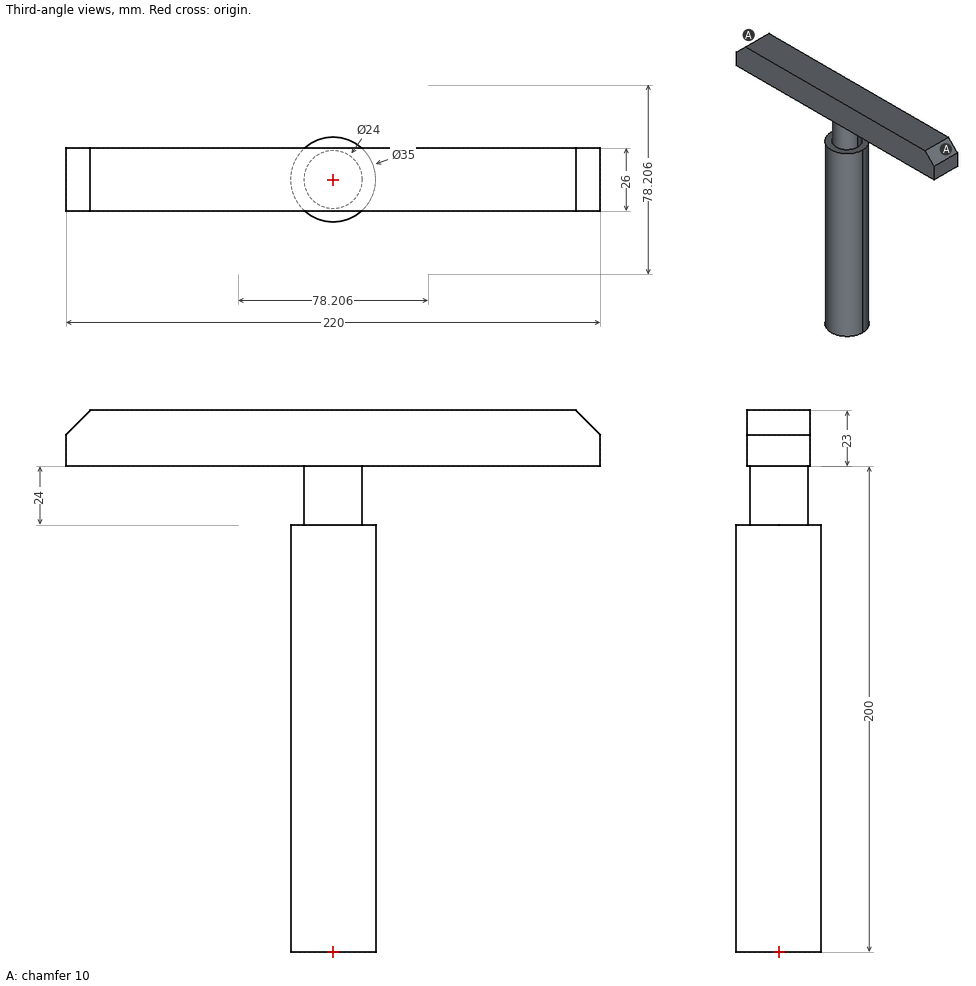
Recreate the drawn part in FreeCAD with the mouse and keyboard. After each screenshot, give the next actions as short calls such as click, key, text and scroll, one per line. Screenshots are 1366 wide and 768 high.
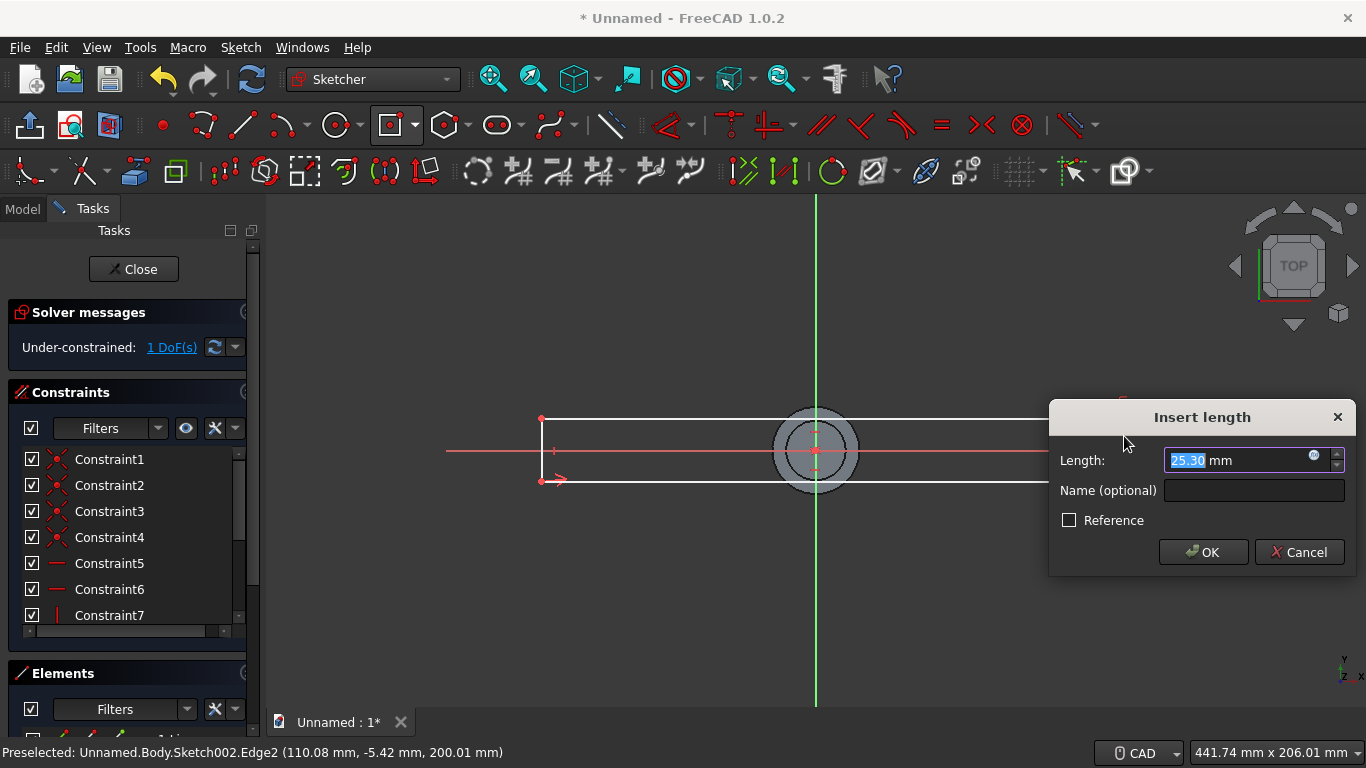
text(26)
key(Return)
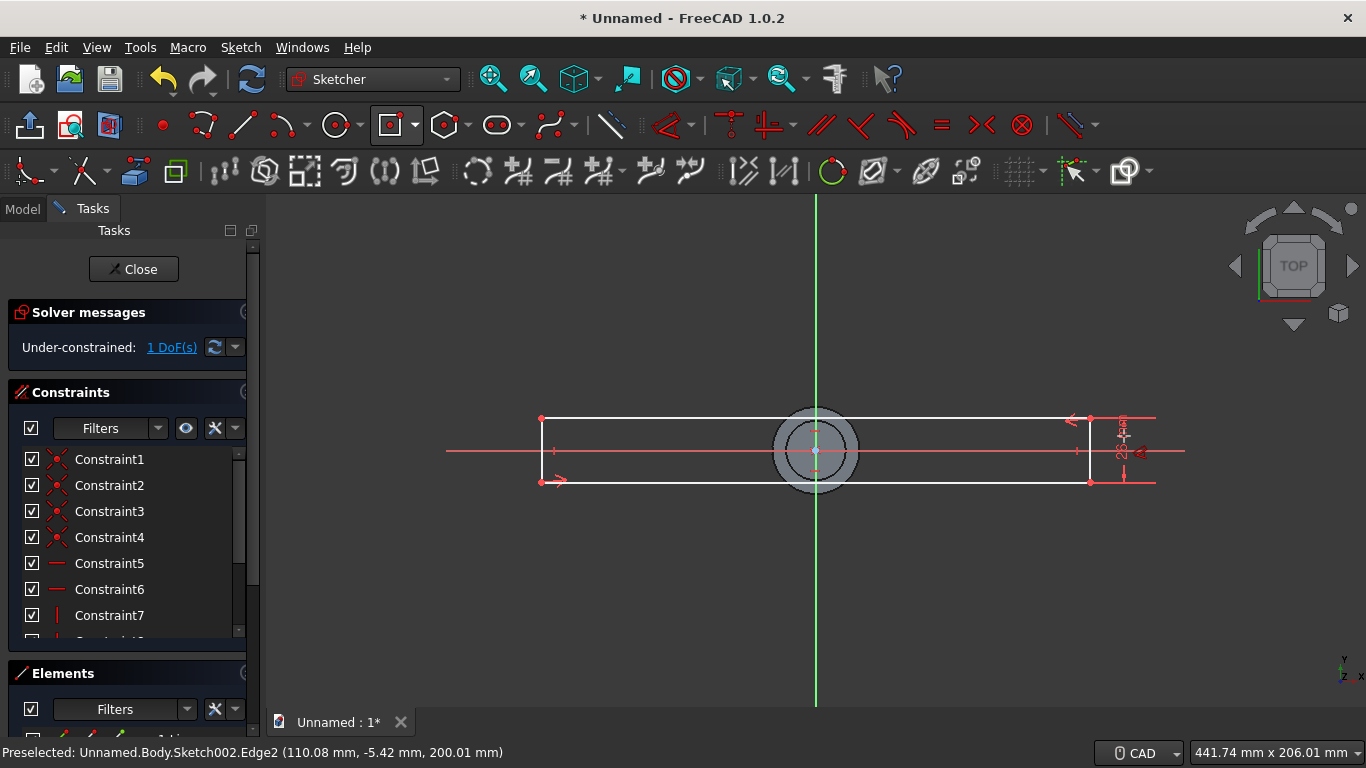
click(706, 483)
click(690, 517)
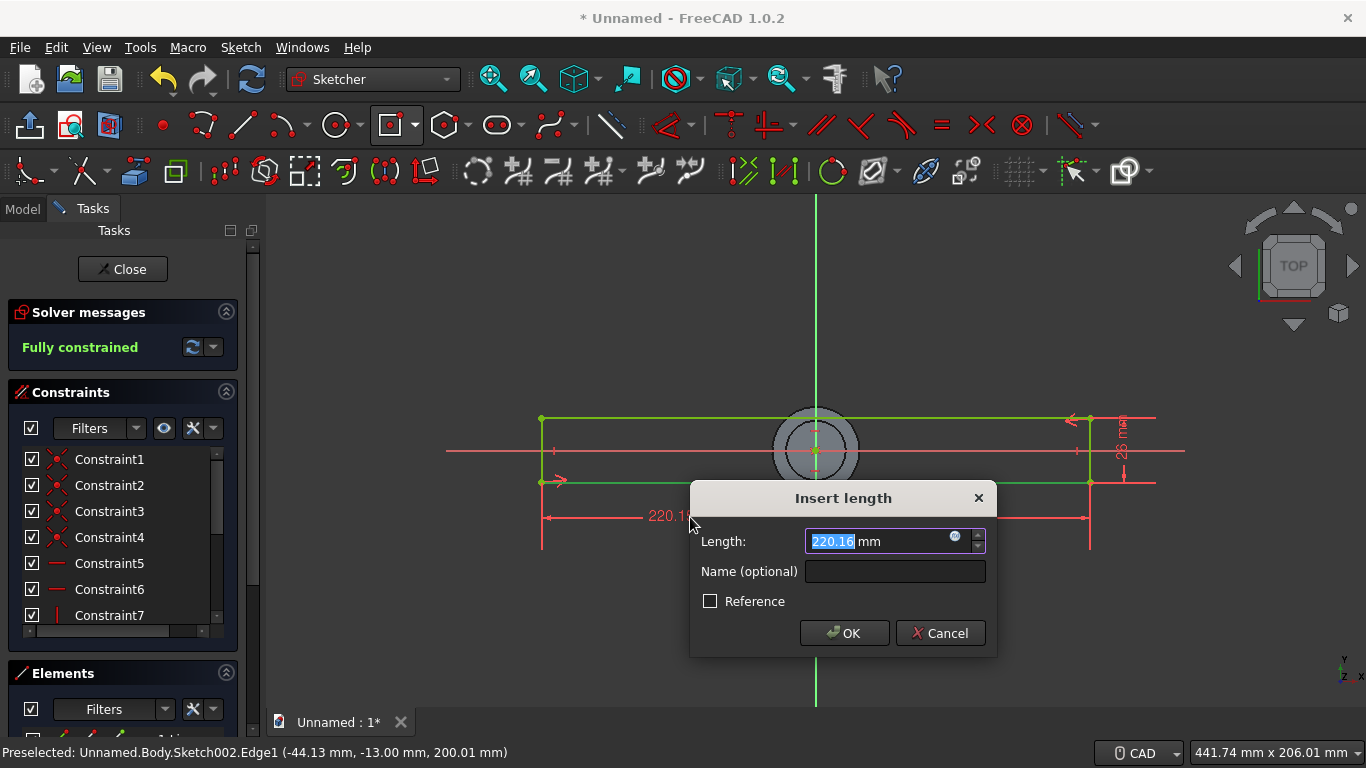
text(220)
key(Return)
key(Escape)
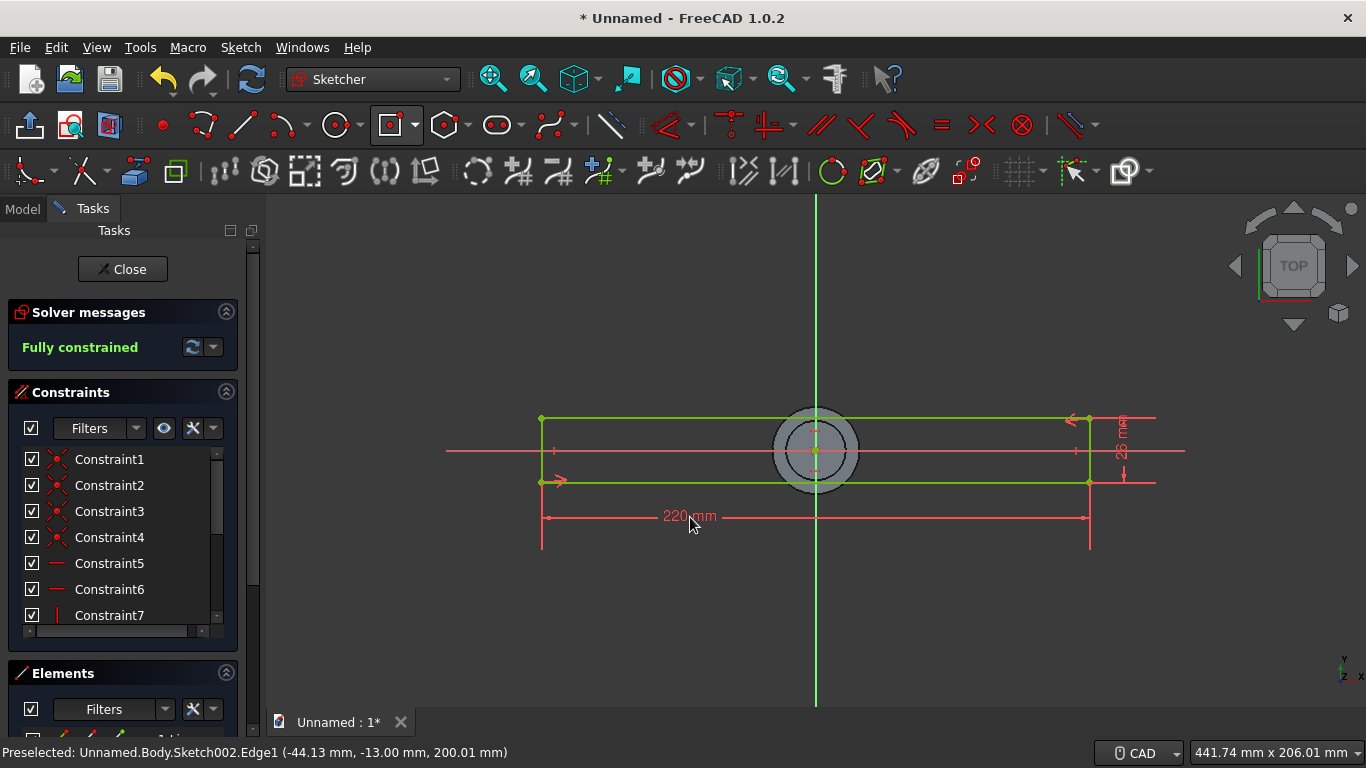
click(123, 269)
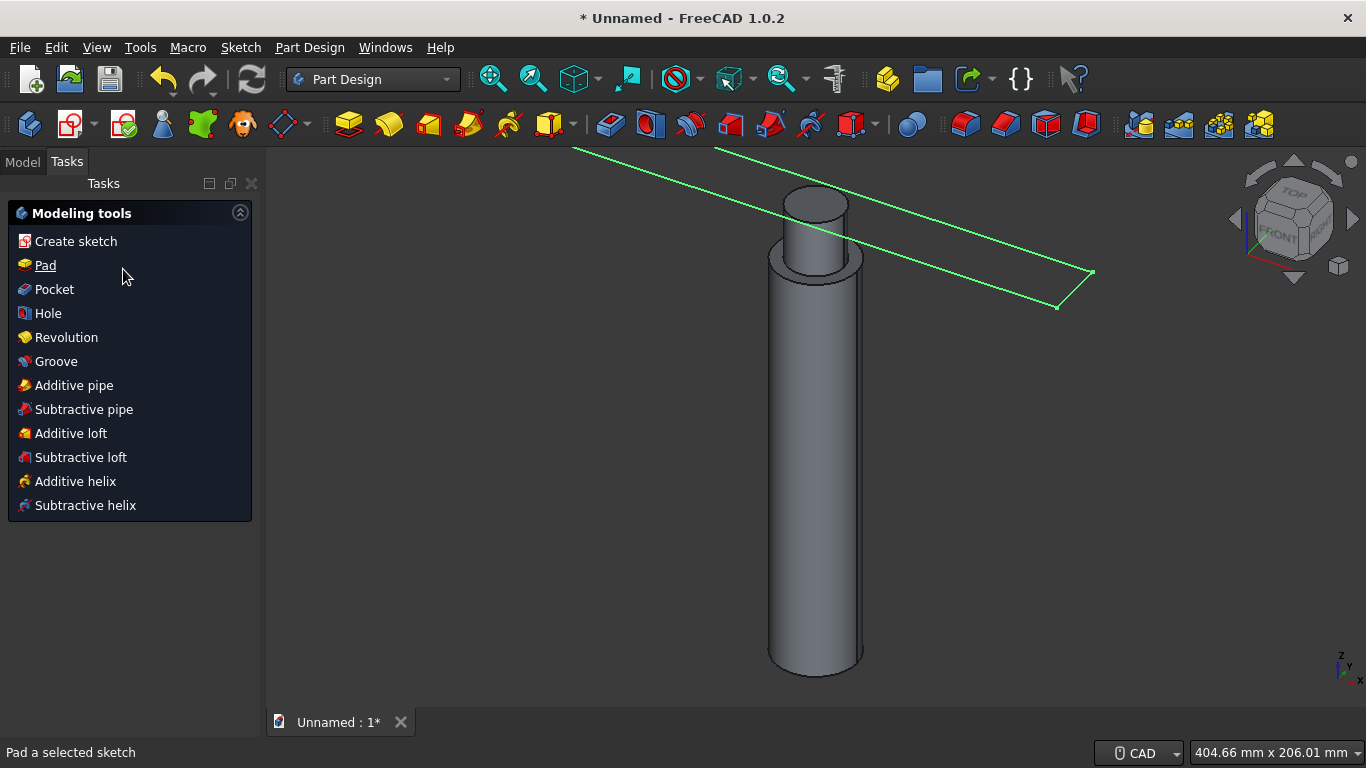
click(350, 124)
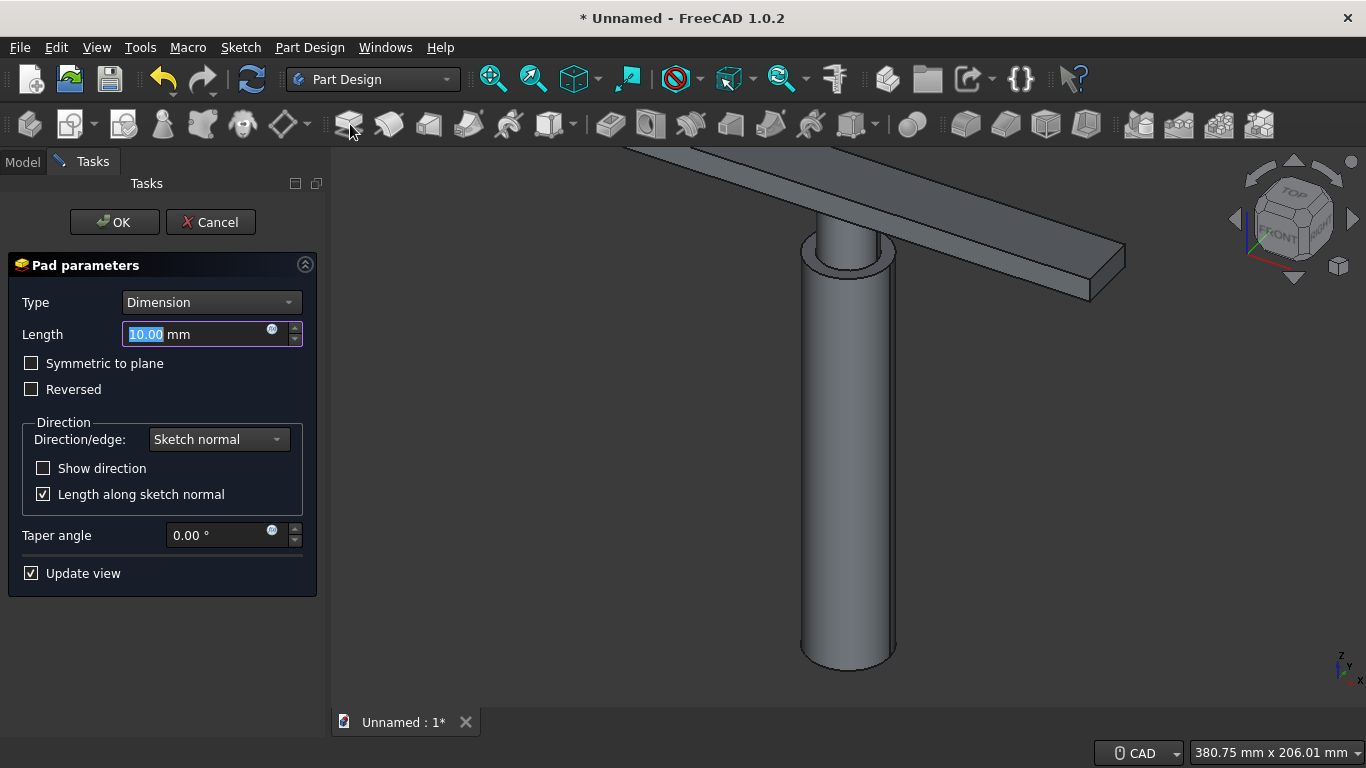
text(23)
key(Tab)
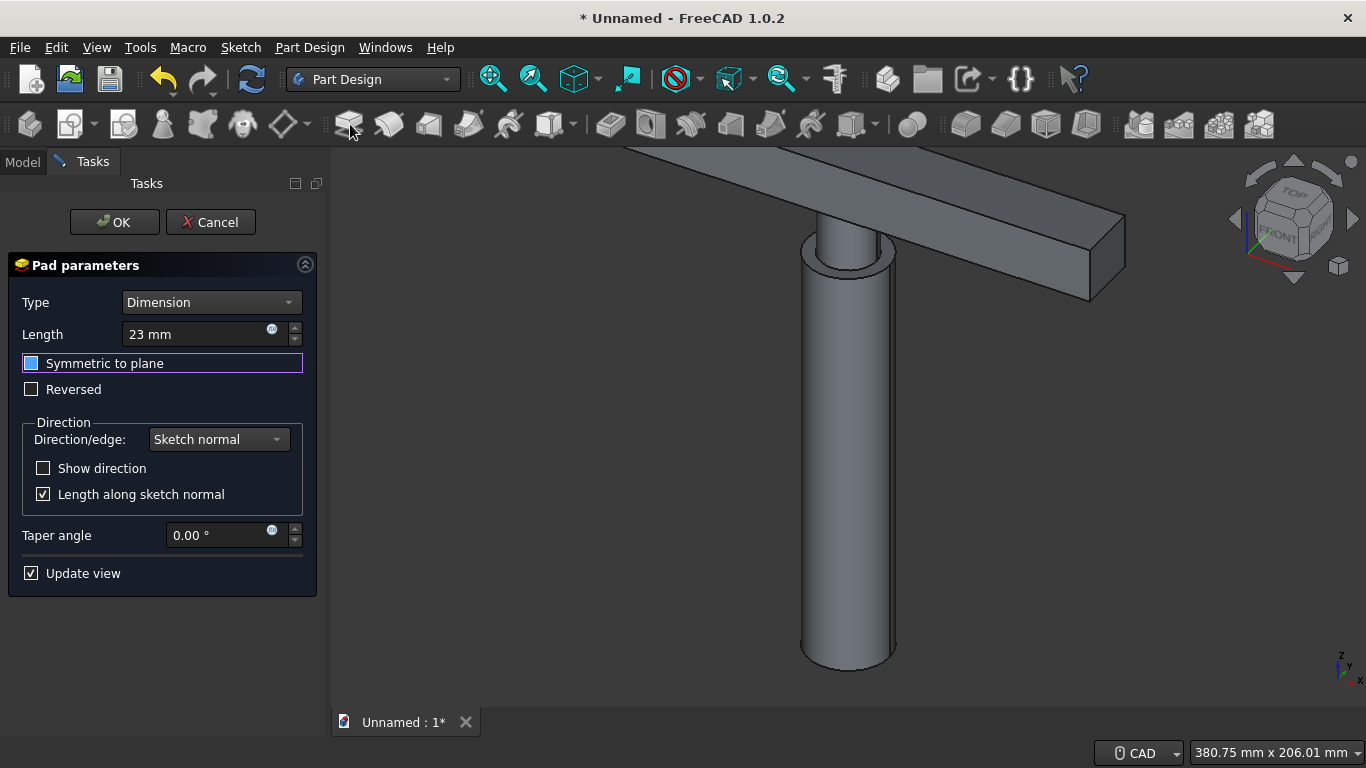
click(115, 222)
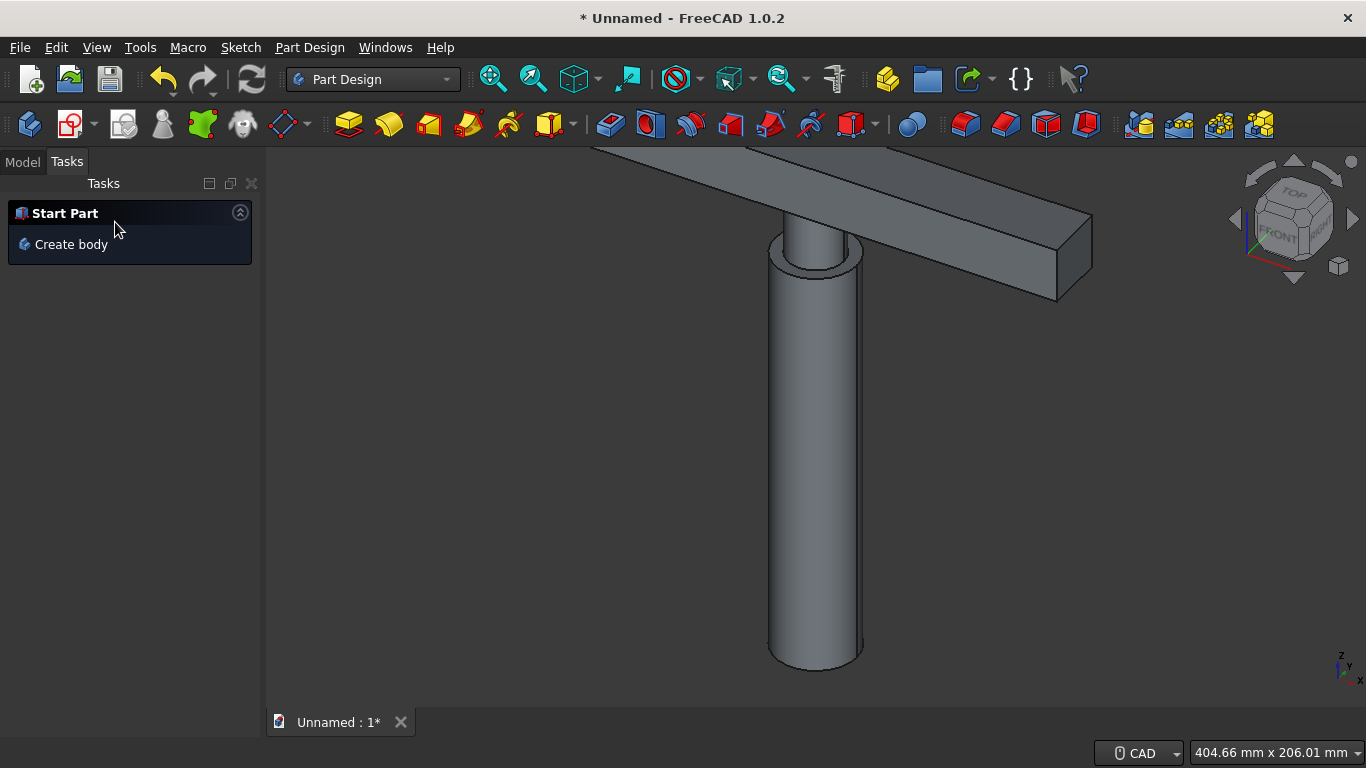
click(494, 80)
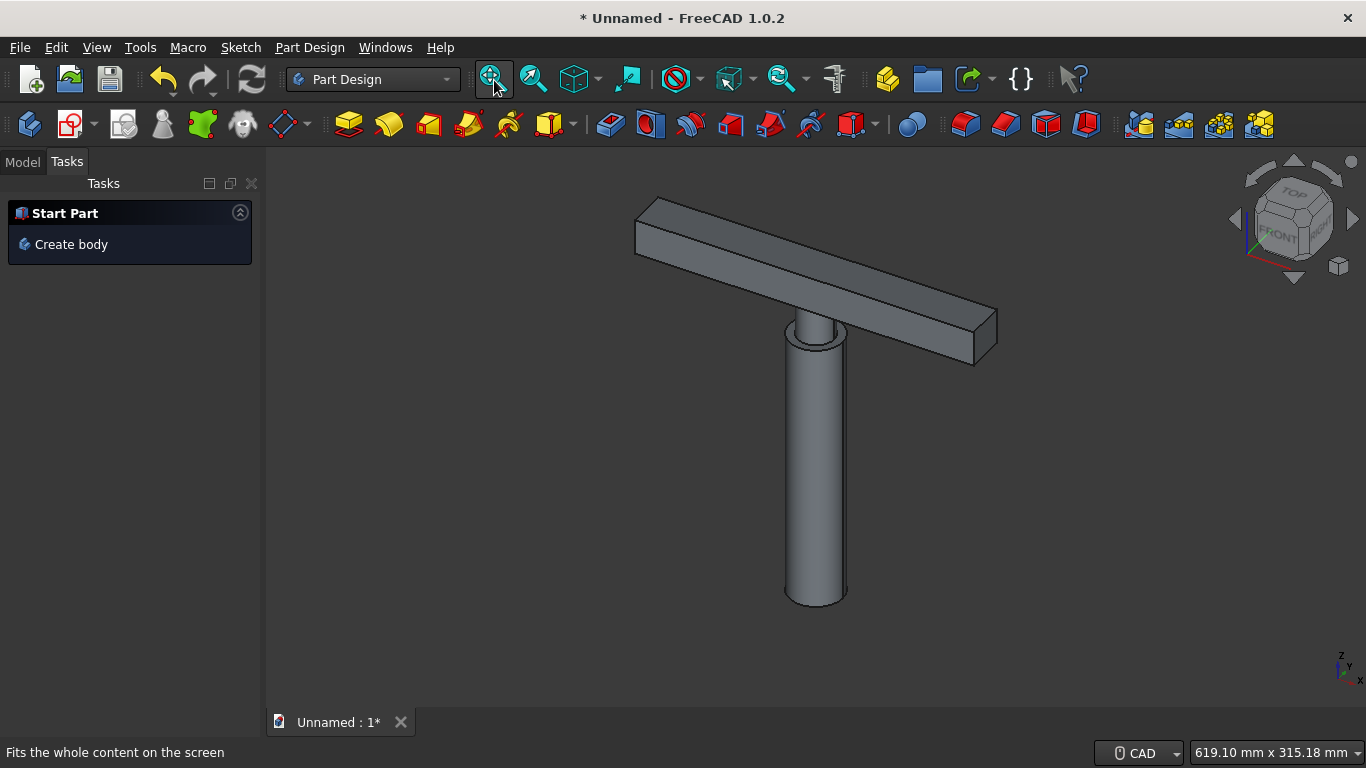
click(985, 320)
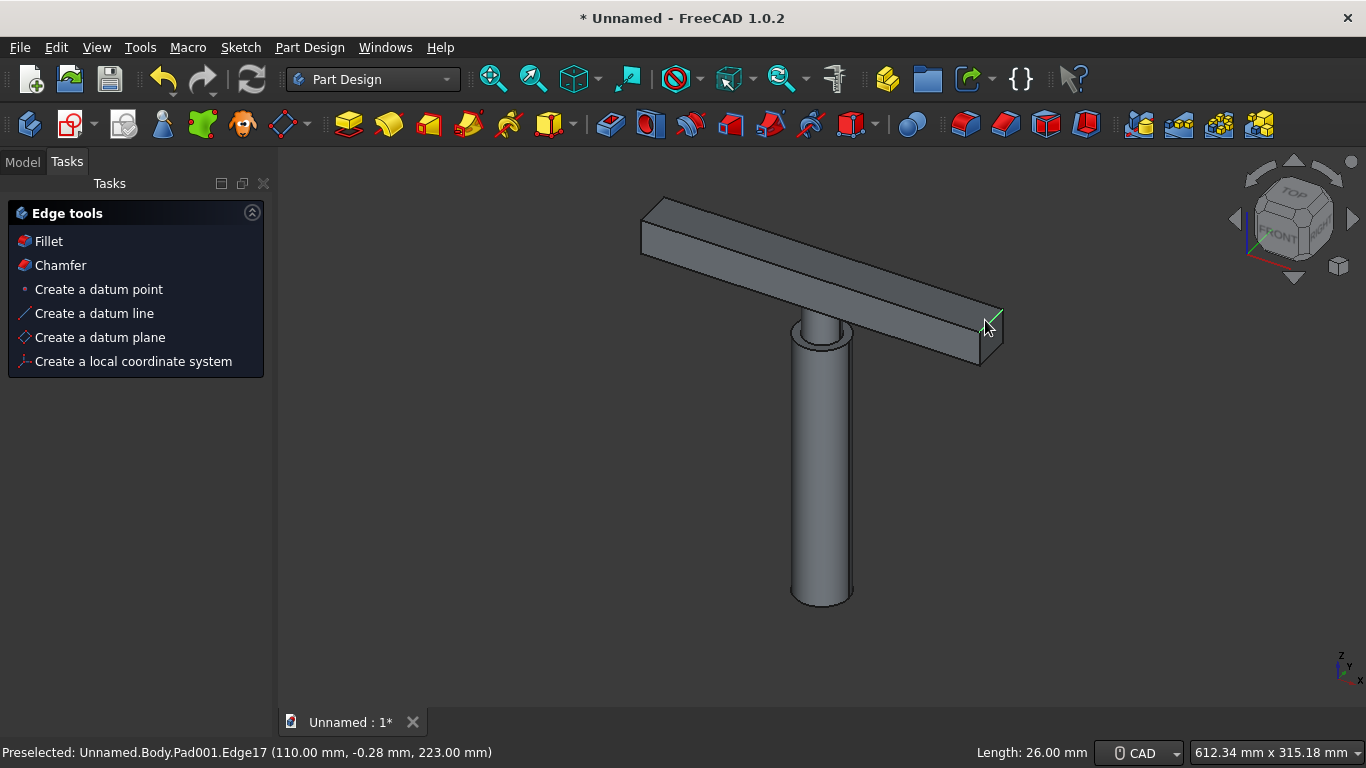
key(0)